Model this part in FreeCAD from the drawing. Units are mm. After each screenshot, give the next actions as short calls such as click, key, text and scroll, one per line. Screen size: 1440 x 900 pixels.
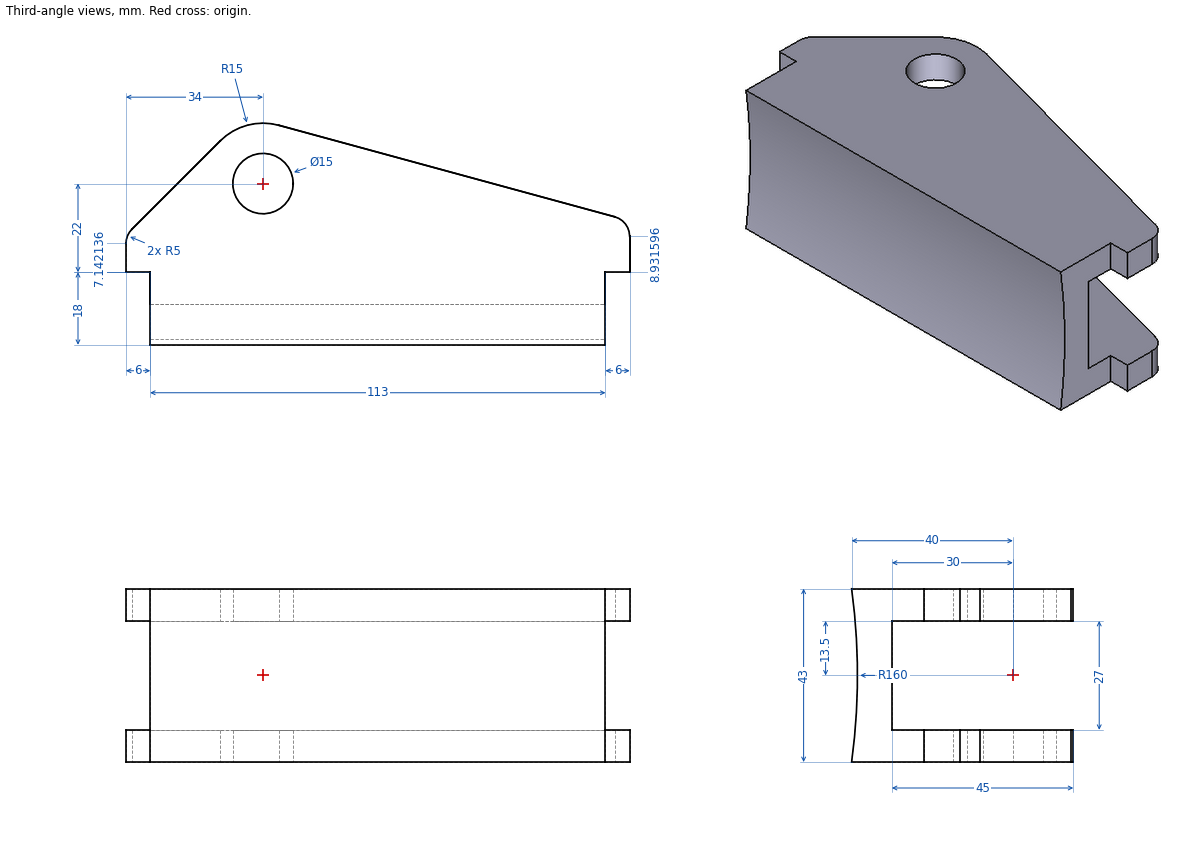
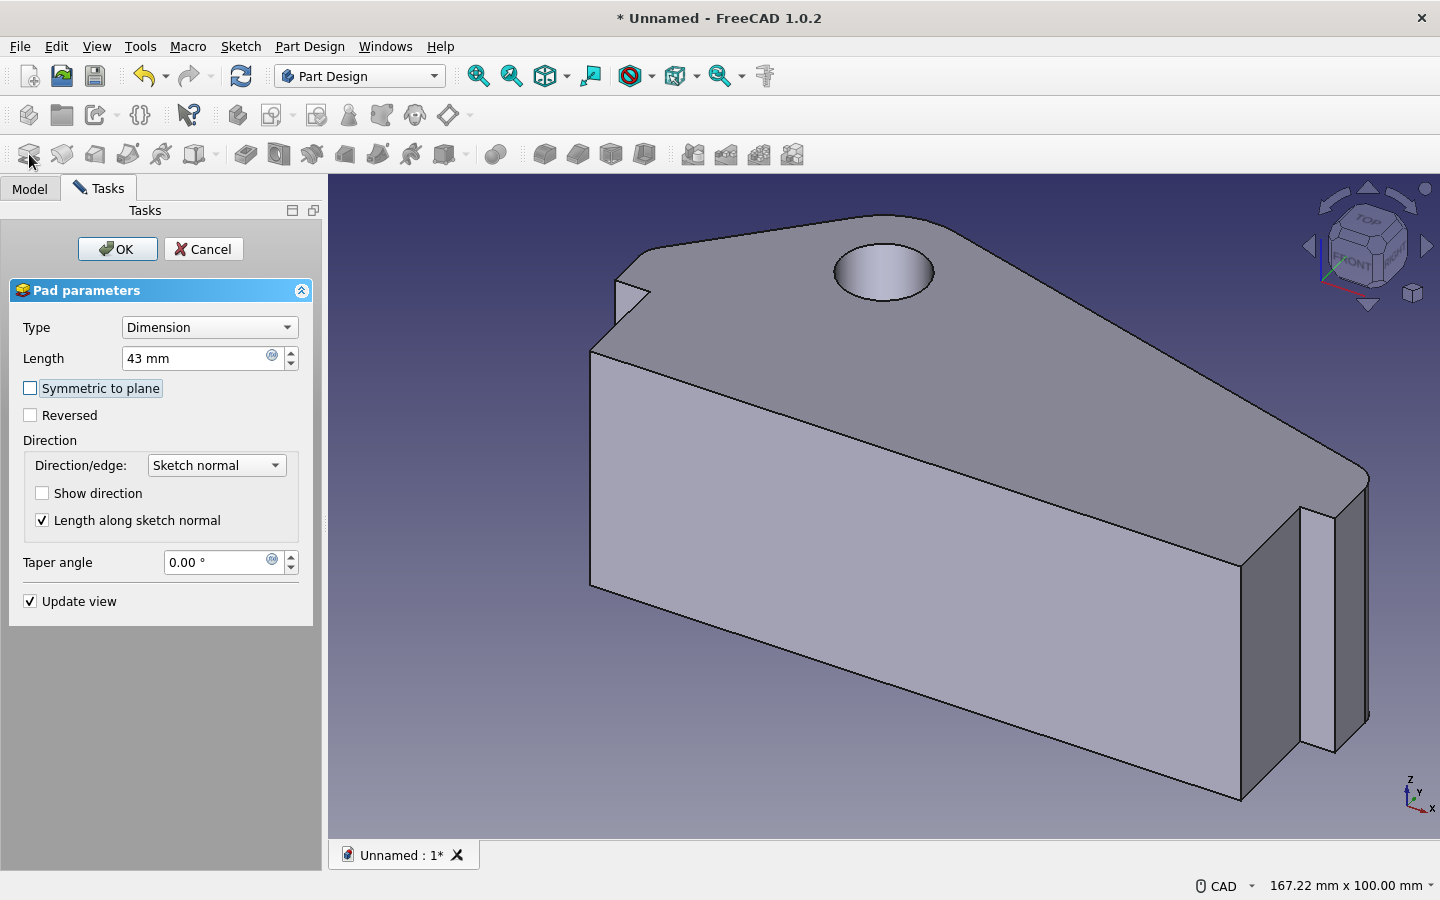
click(31, 388)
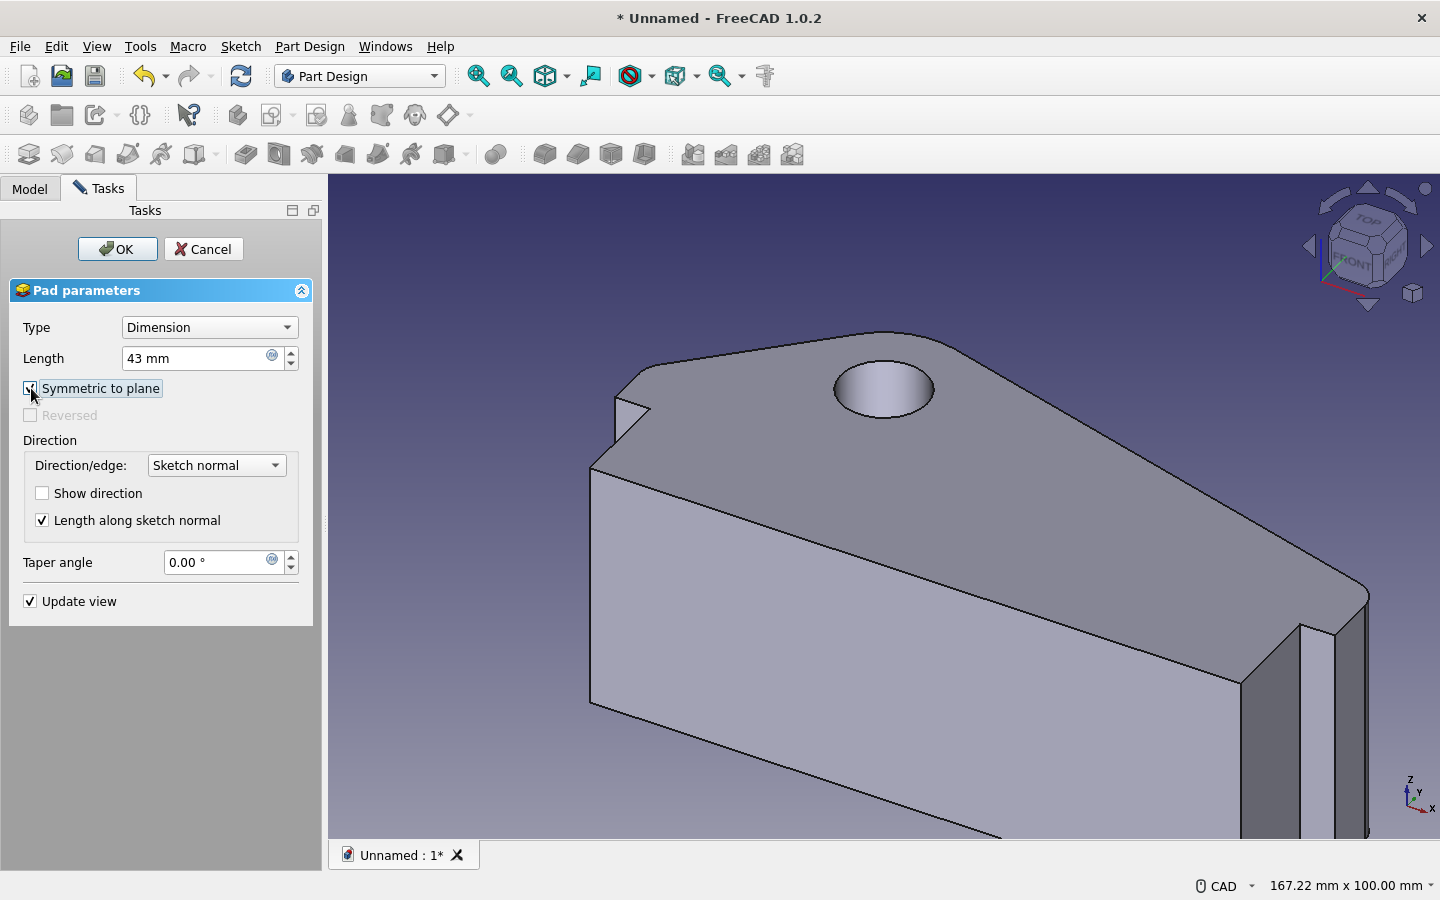
click(118, 249)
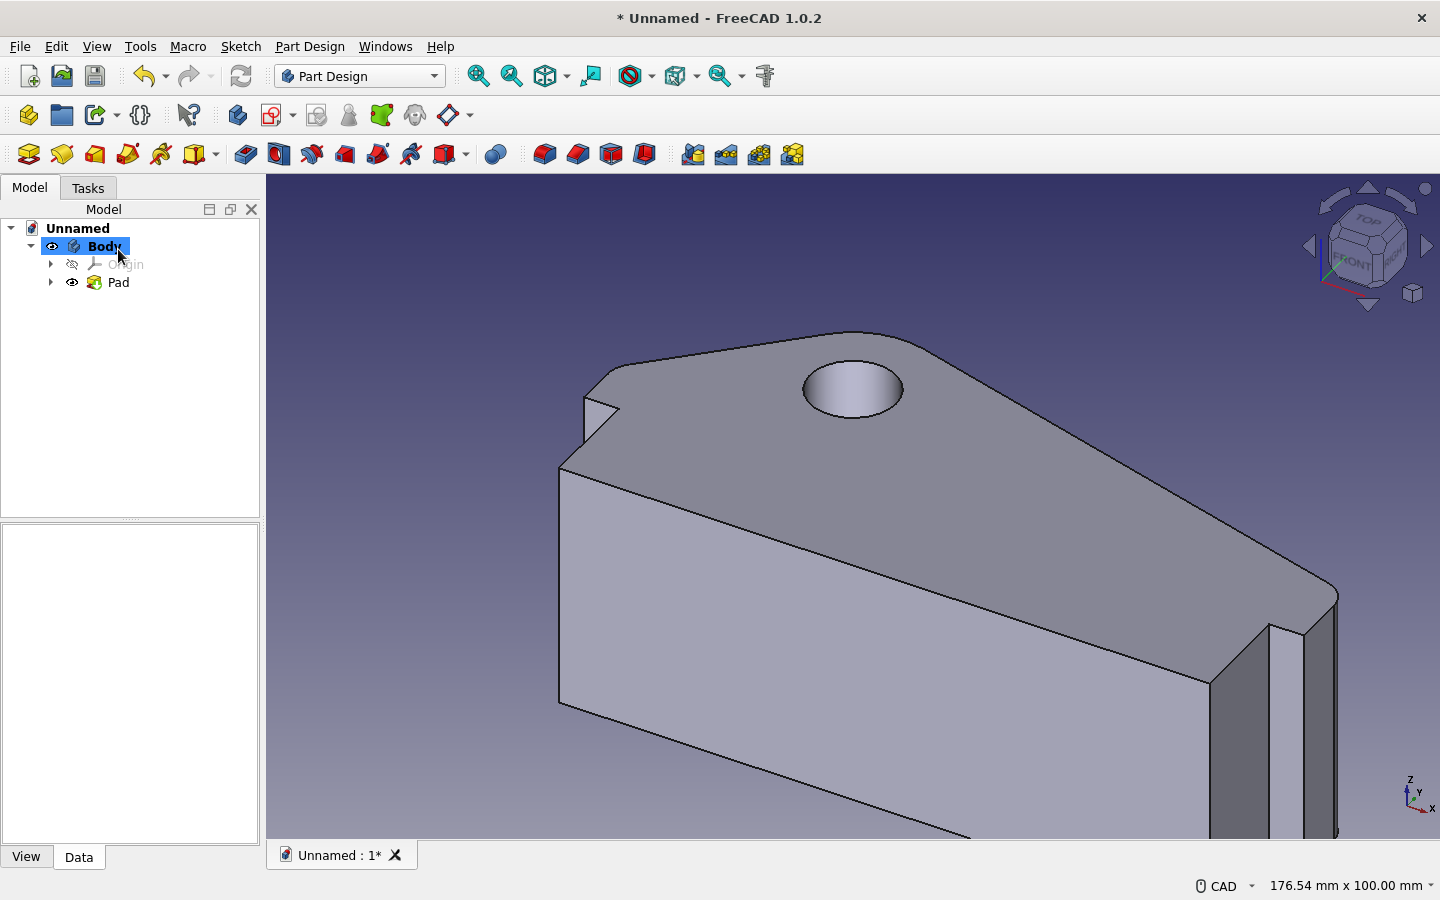
click(479, 76)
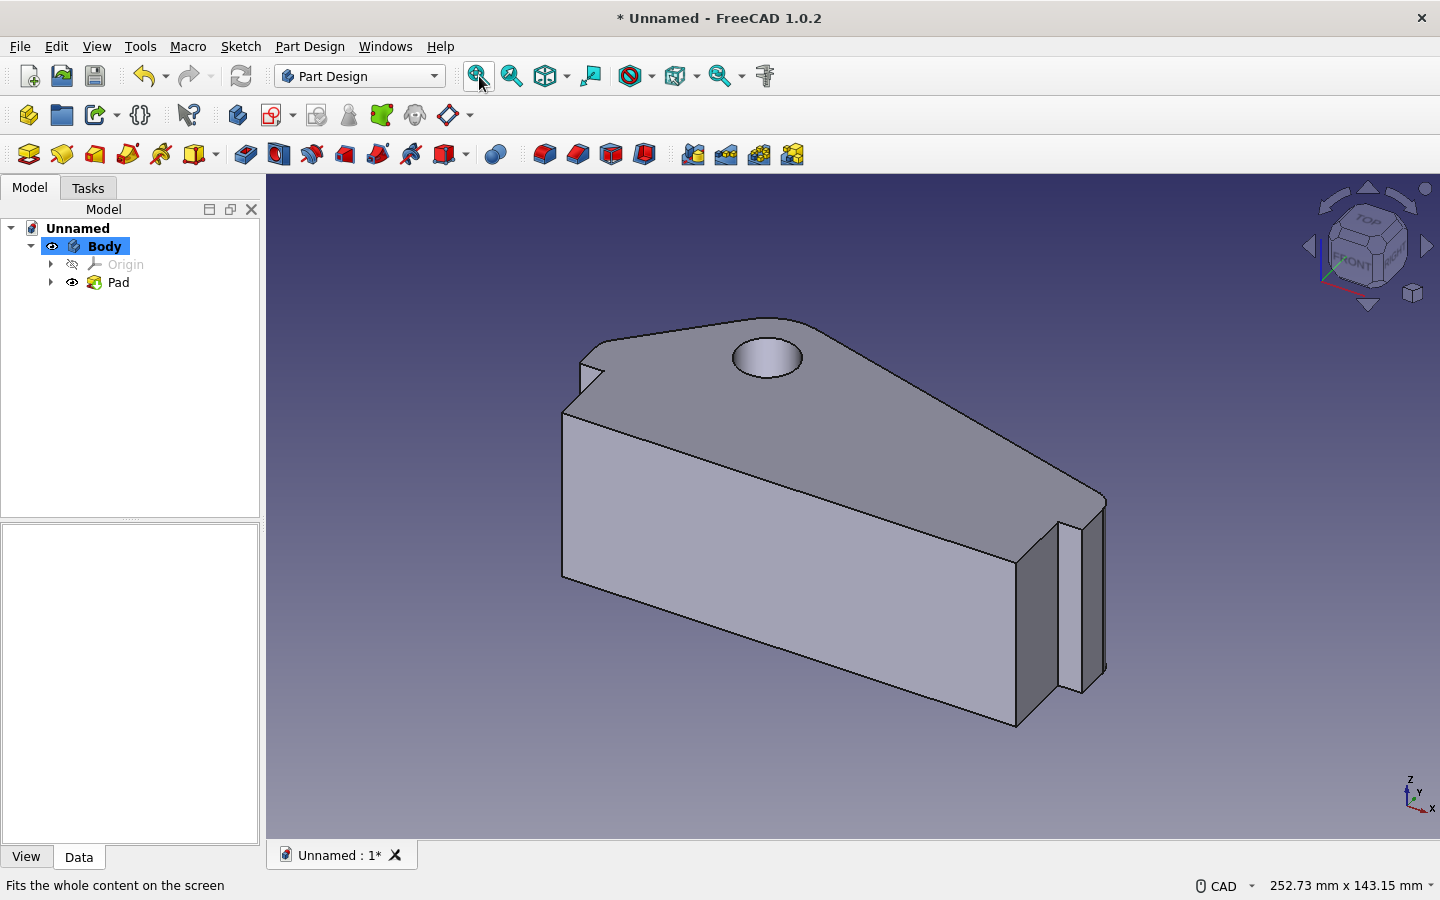
click(1037, 577)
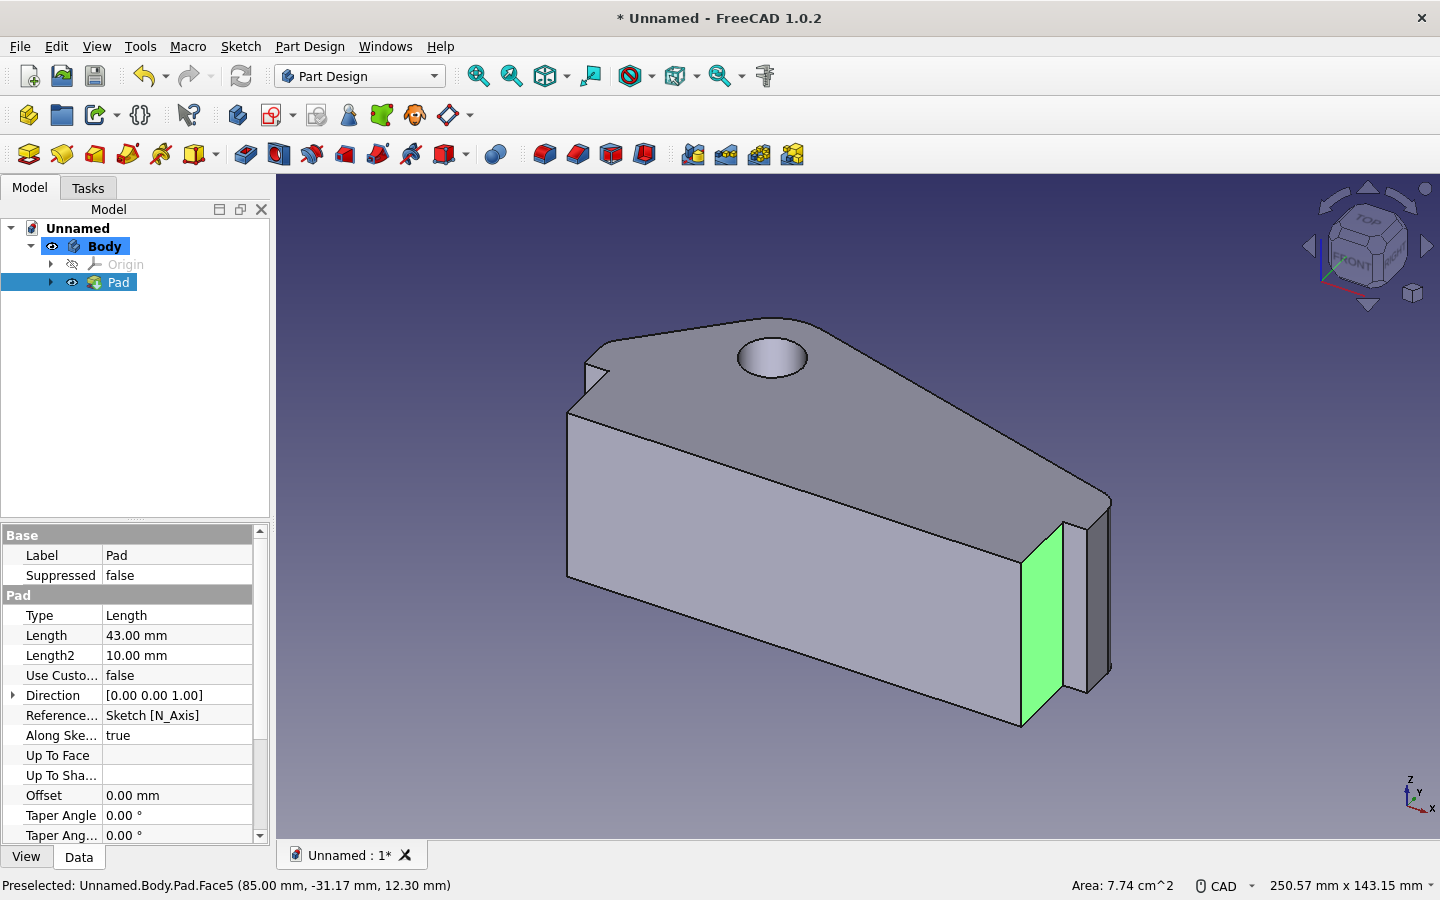
click(270, 116)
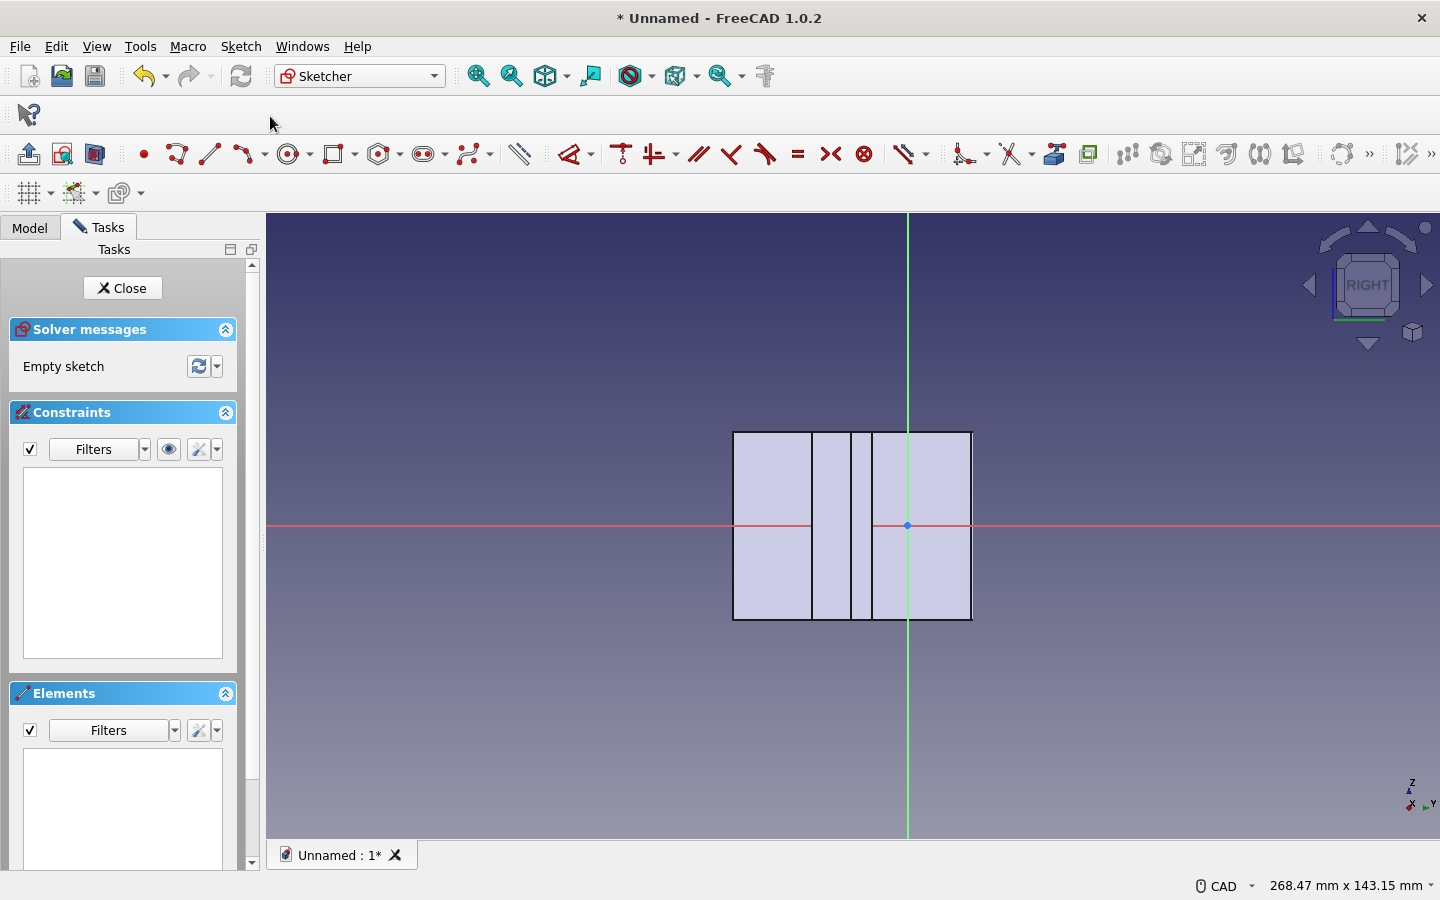
key(q)
key(s)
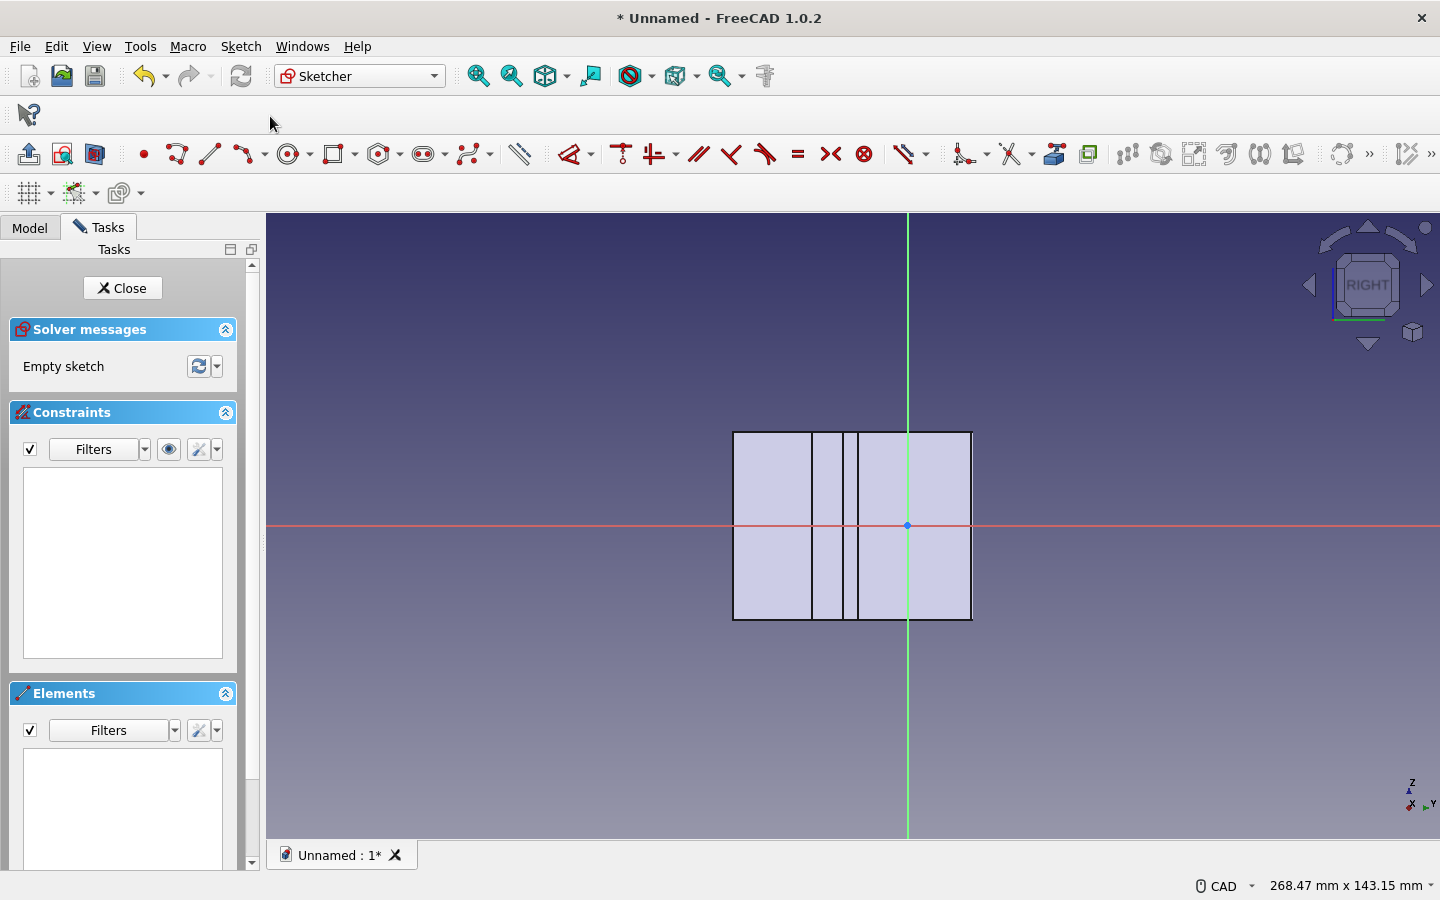
scroll(909, 526, up, 4)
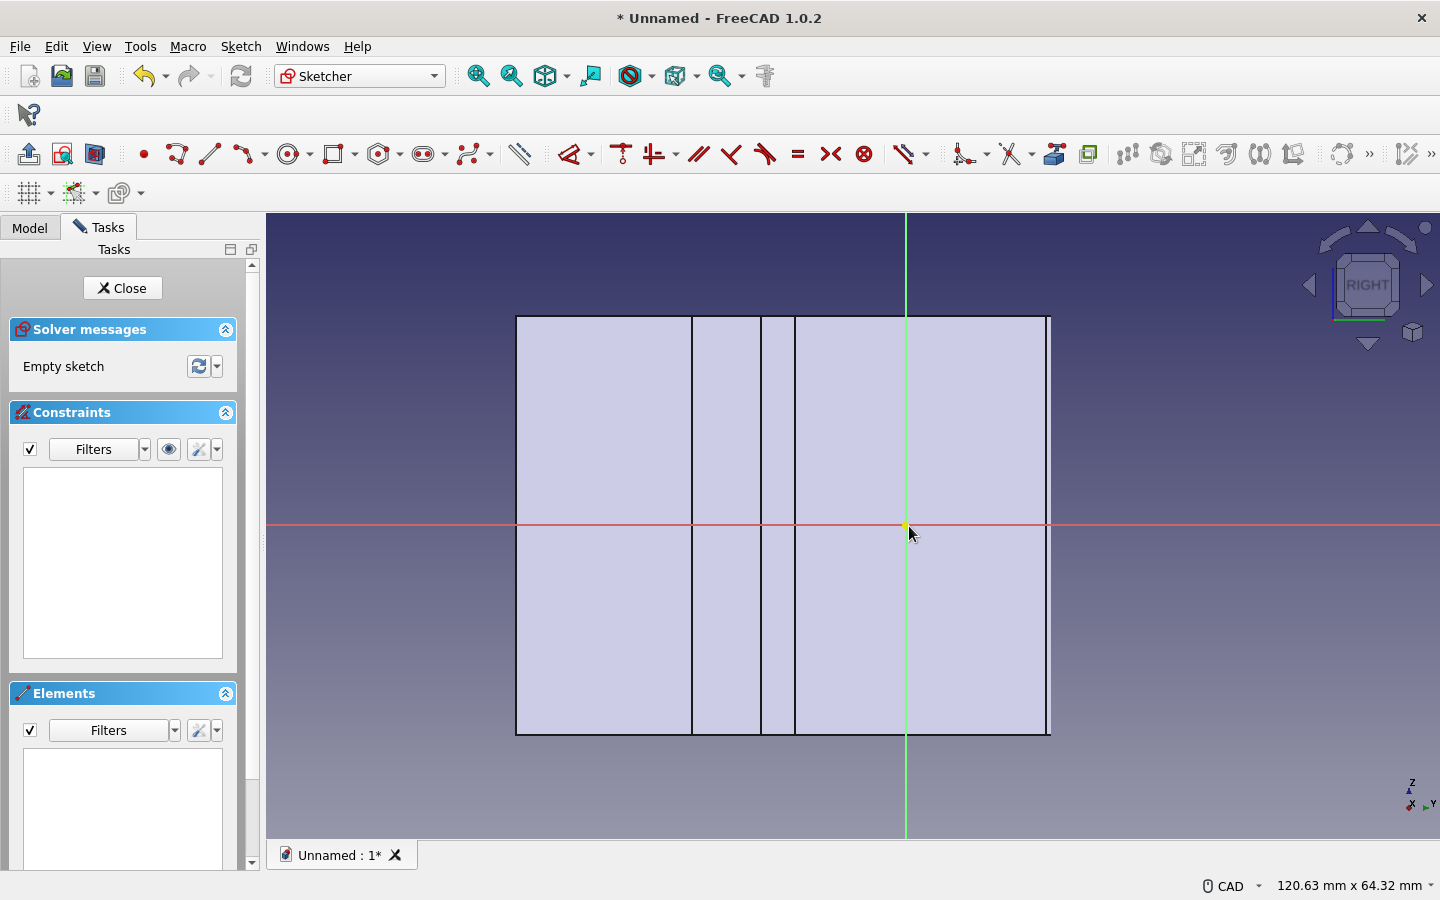
click(332, 154)